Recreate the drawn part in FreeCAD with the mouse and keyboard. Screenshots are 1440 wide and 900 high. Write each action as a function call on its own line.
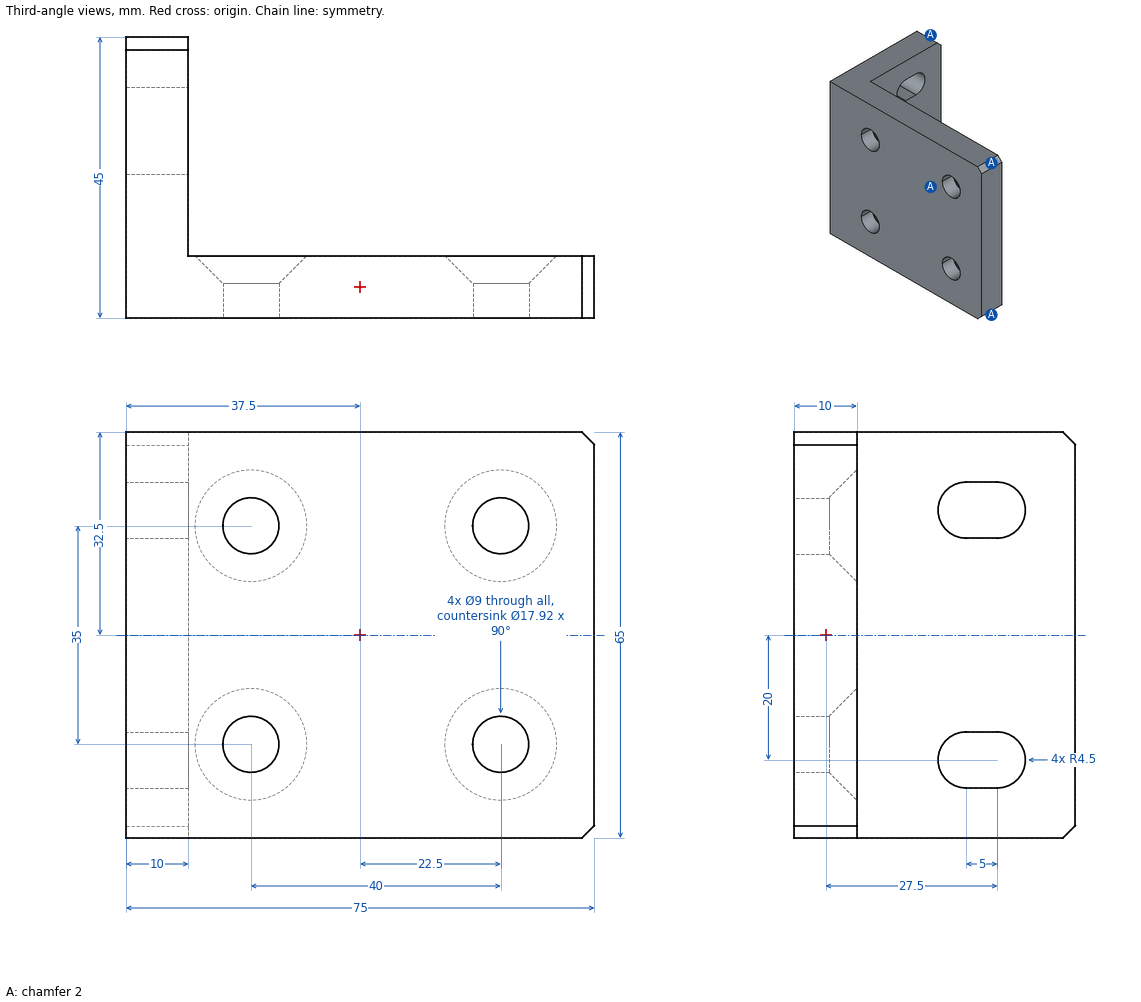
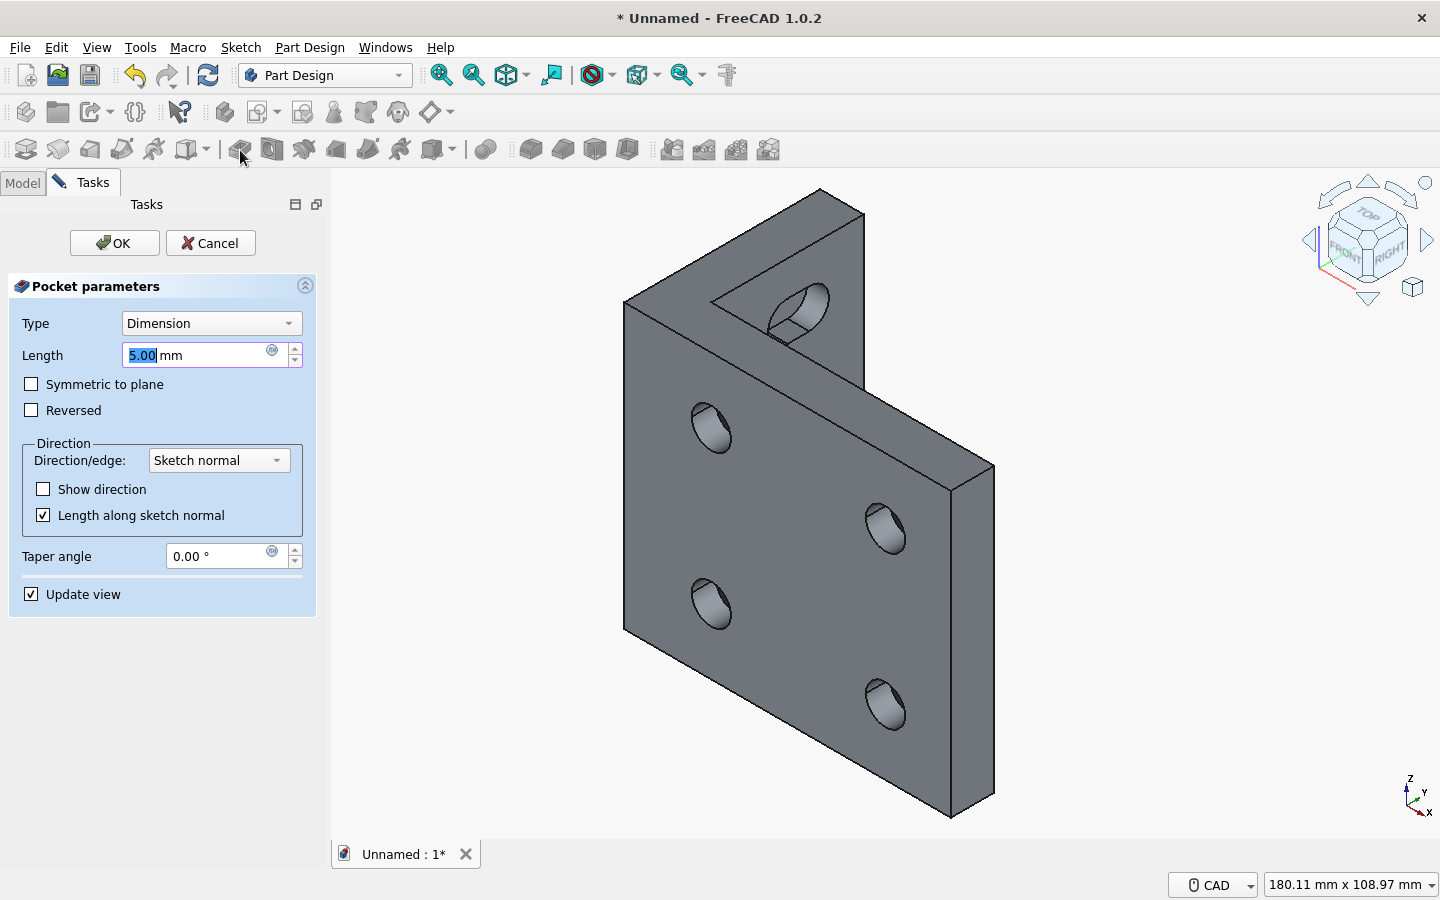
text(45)
key(Tab)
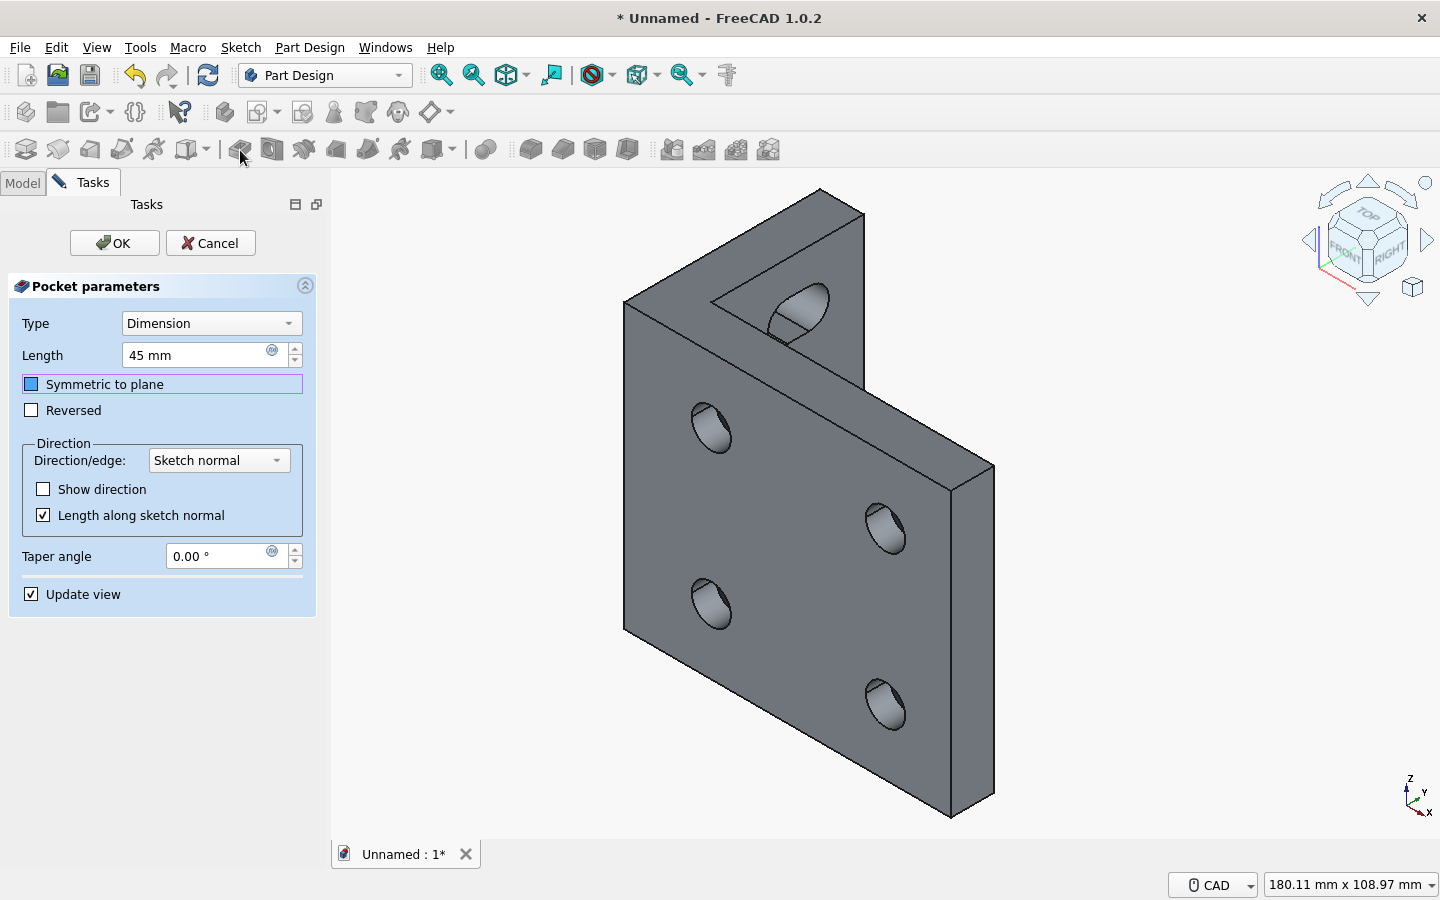
click(115, 243)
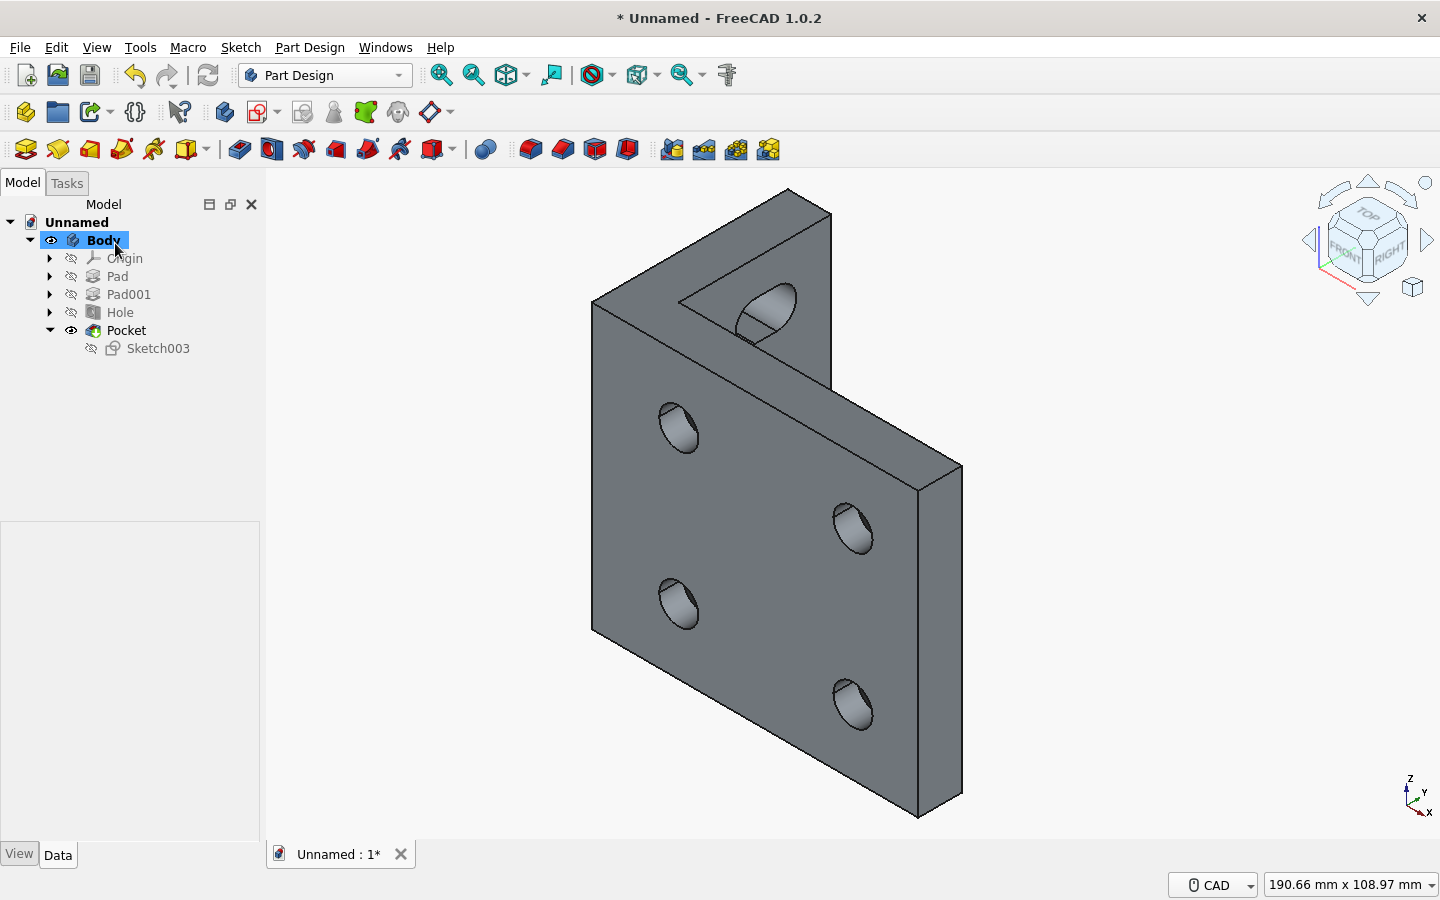
click(940, 477)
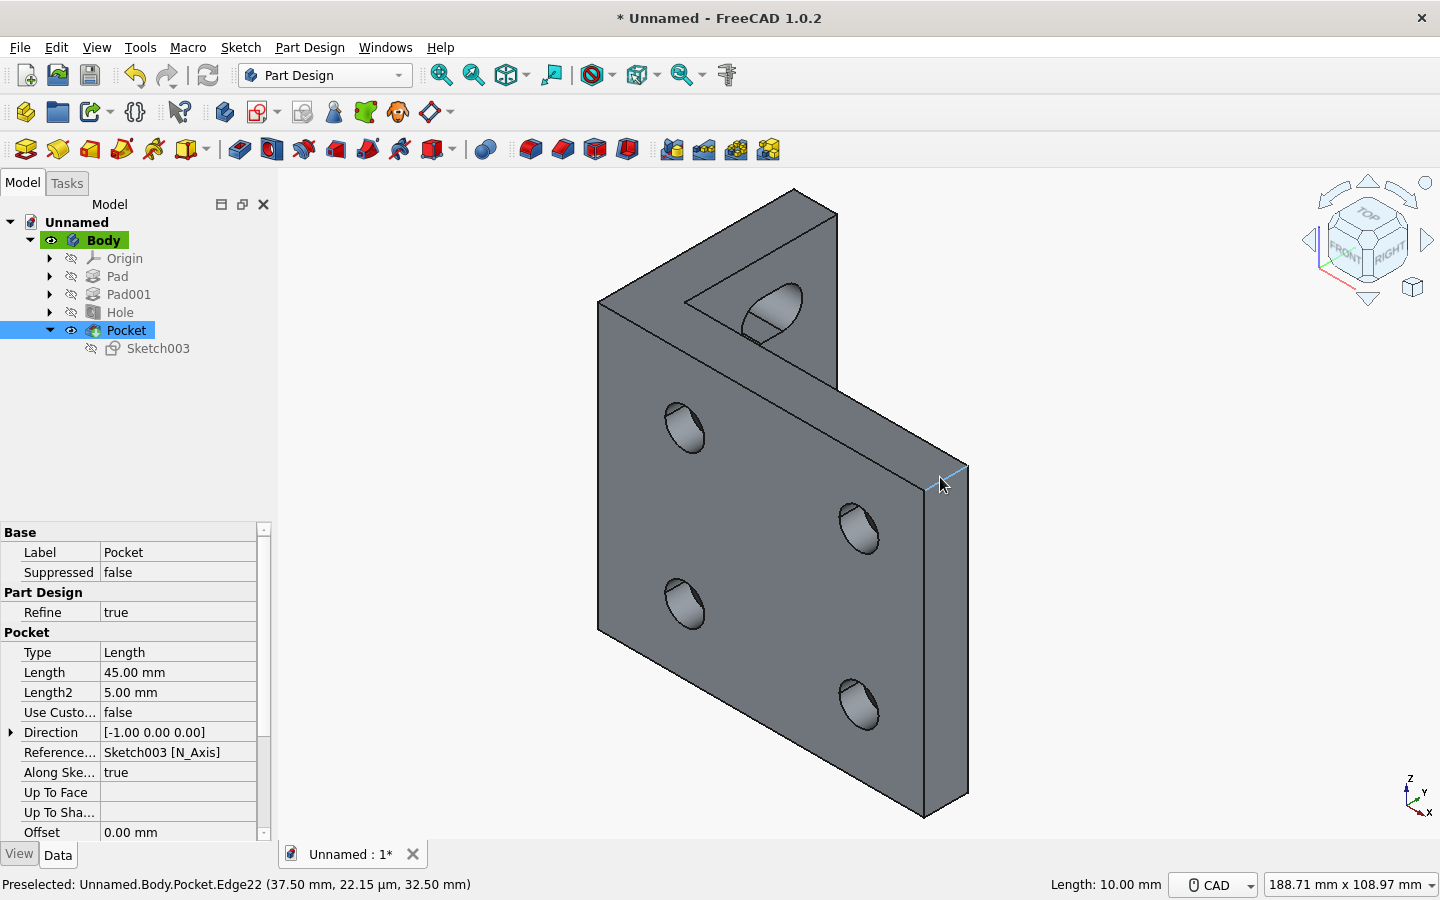
key(2)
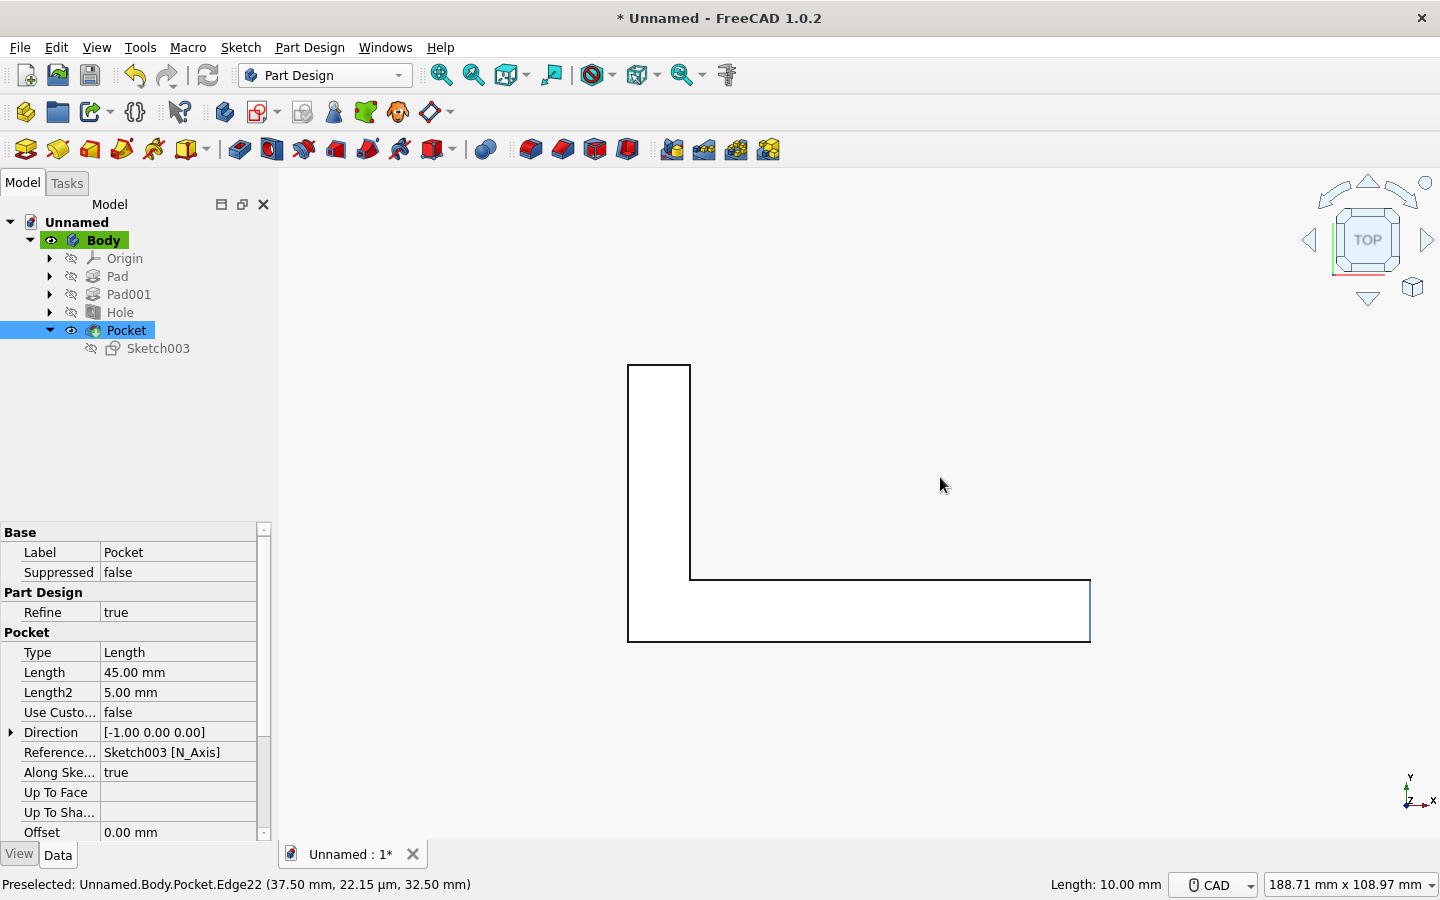
key(v)
key(f)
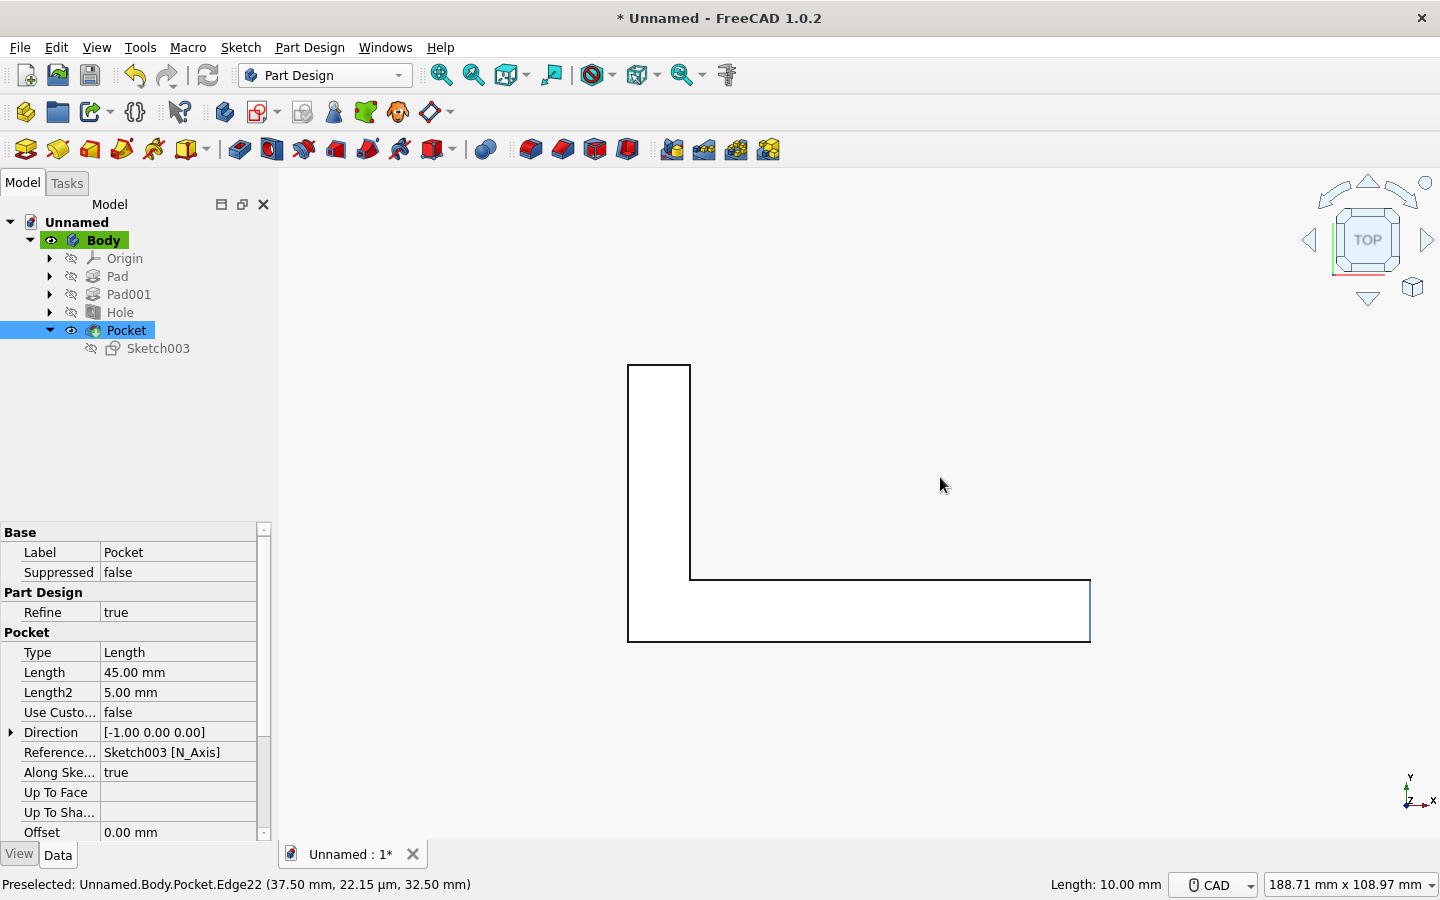
click(659, 364, ctrl)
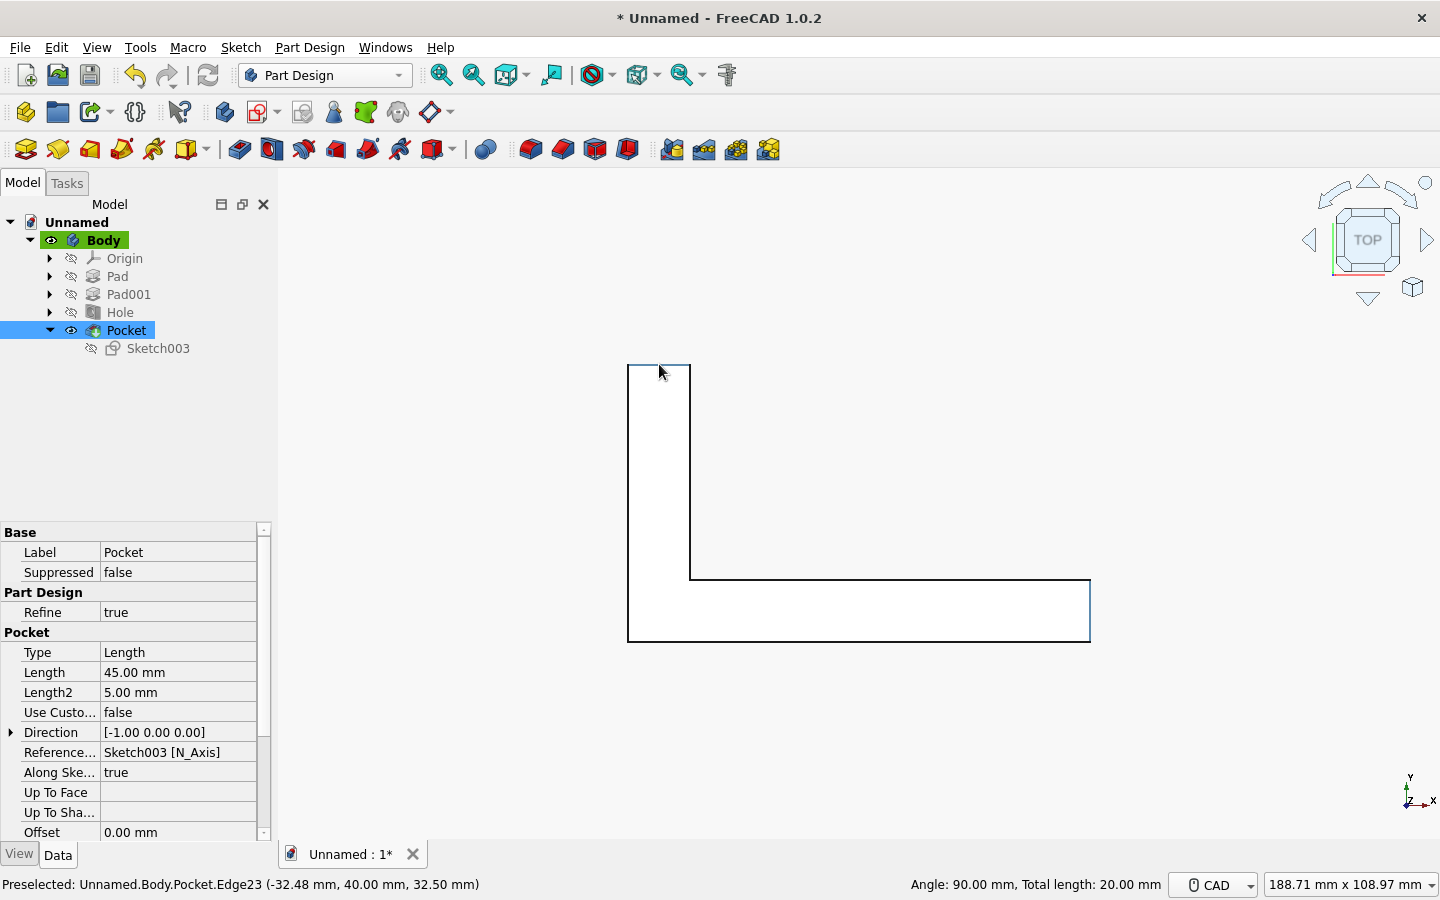
key(0)